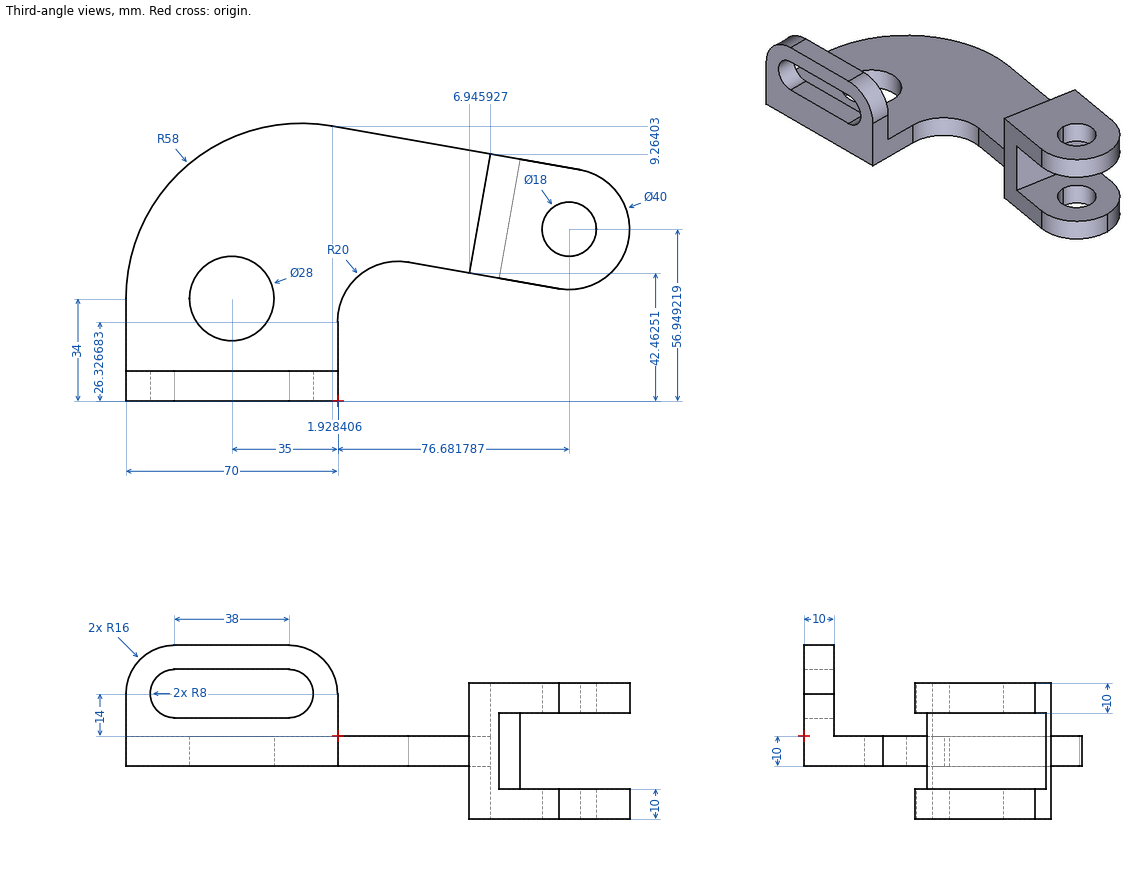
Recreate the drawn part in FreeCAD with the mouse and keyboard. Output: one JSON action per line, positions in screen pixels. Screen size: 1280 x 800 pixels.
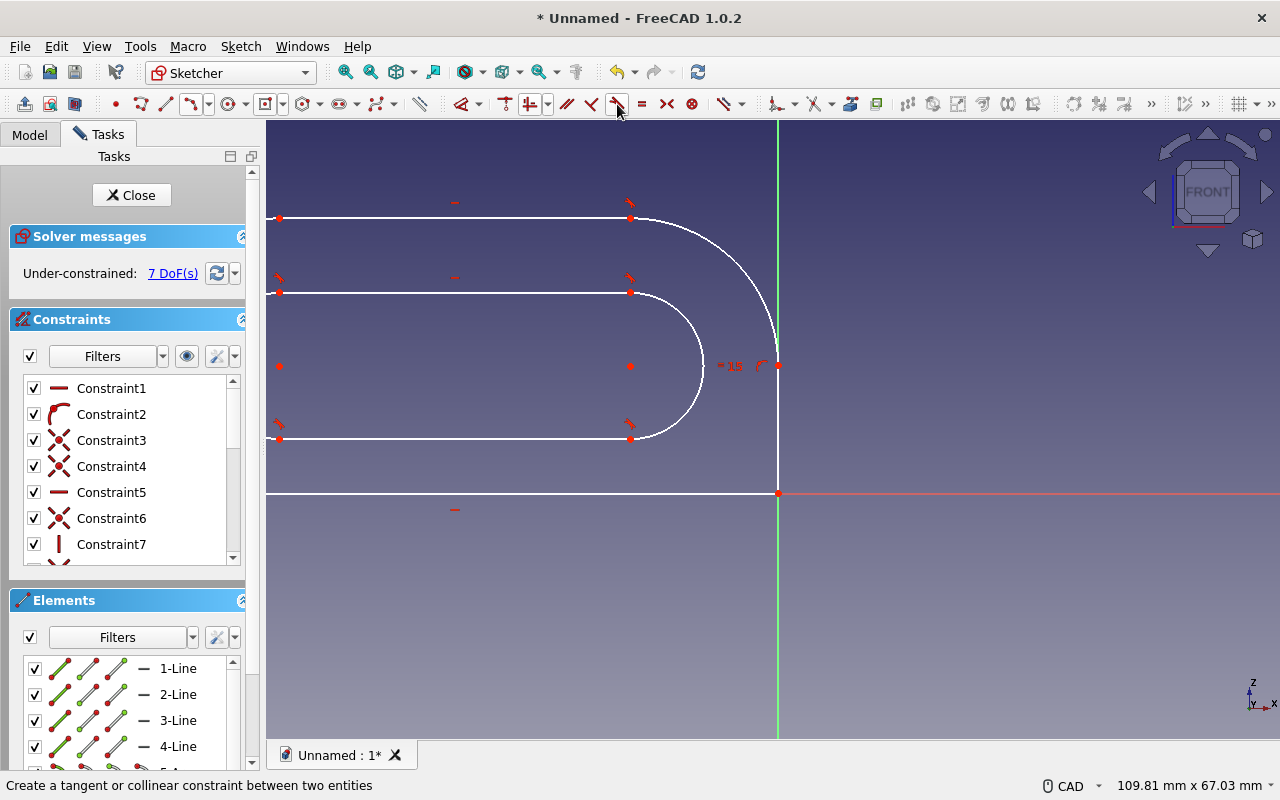
{"action": "left_click", "coordinate": [385, 218]}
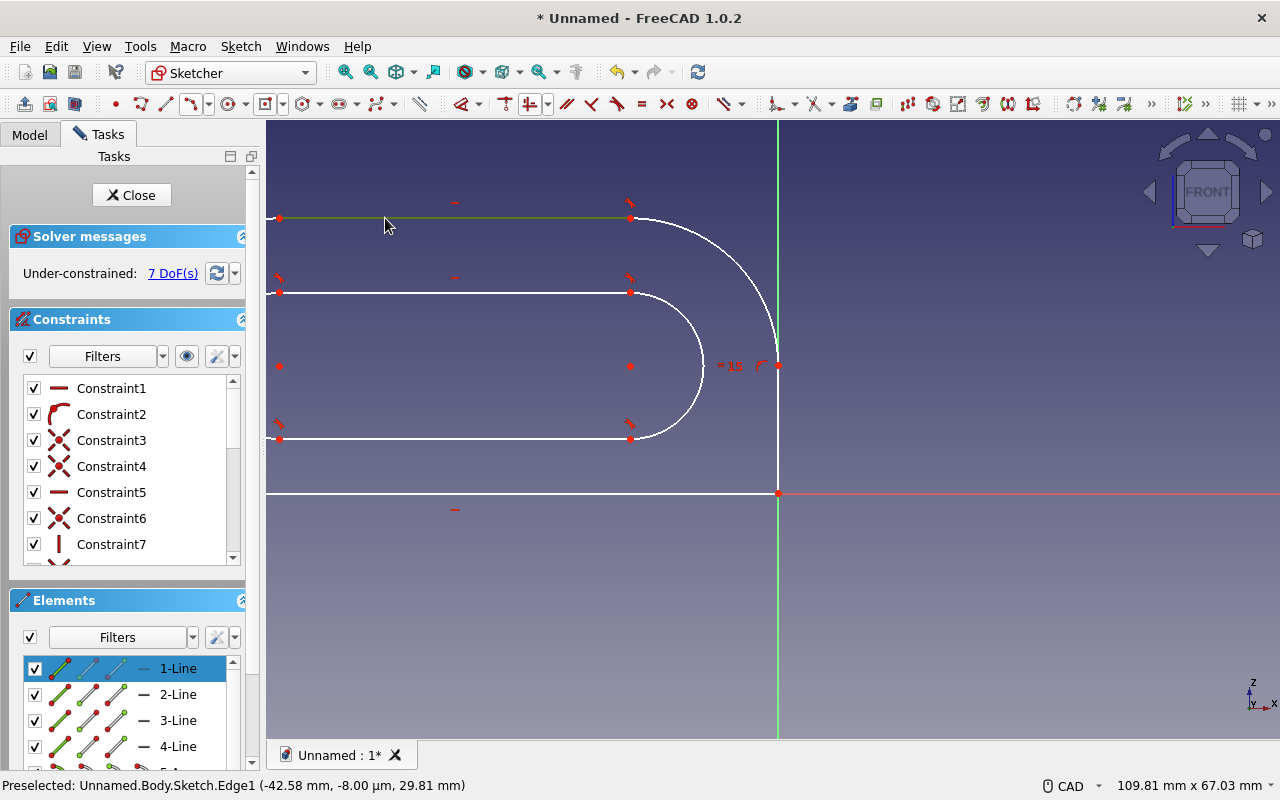
{"action": "scroll", "coordinate": [1115, 581], "scroll_direction": "down", "scroll_amount": 2}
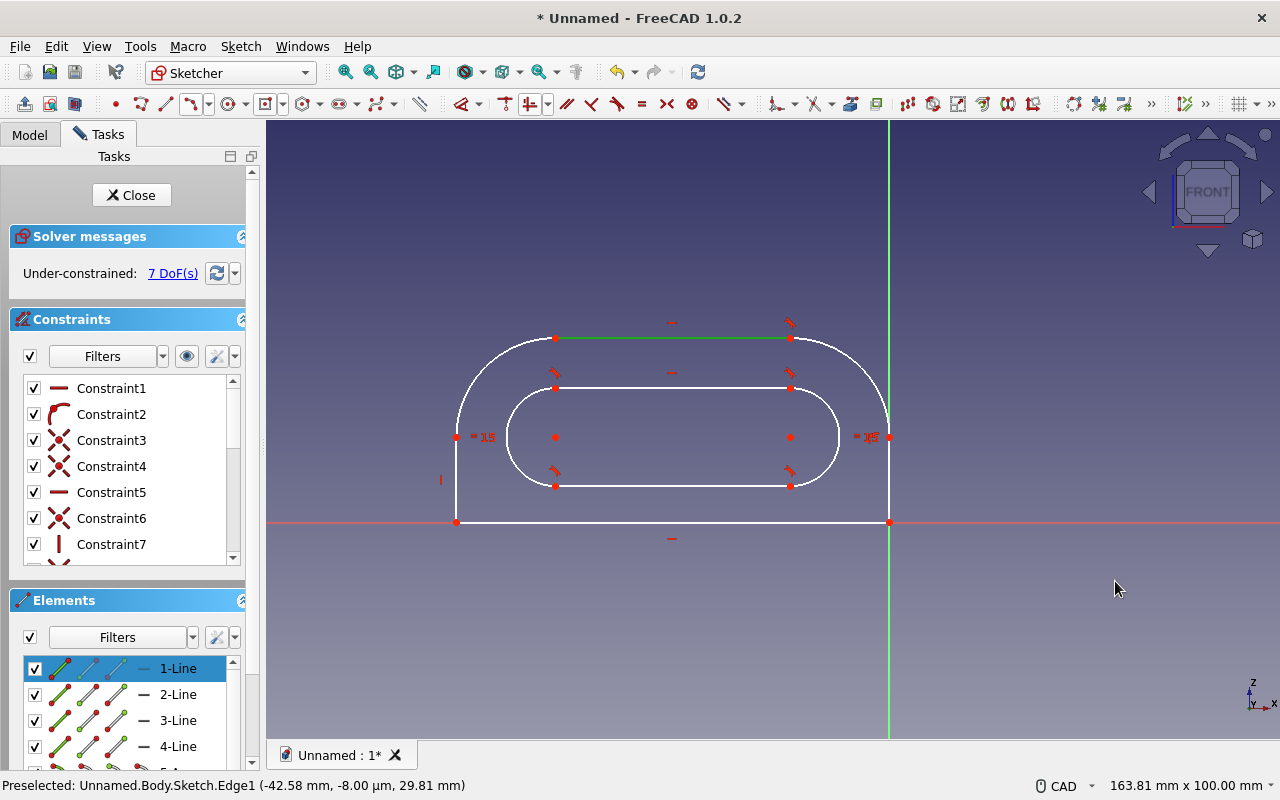
{"action": "left_click", "coordinate": [511, 349]}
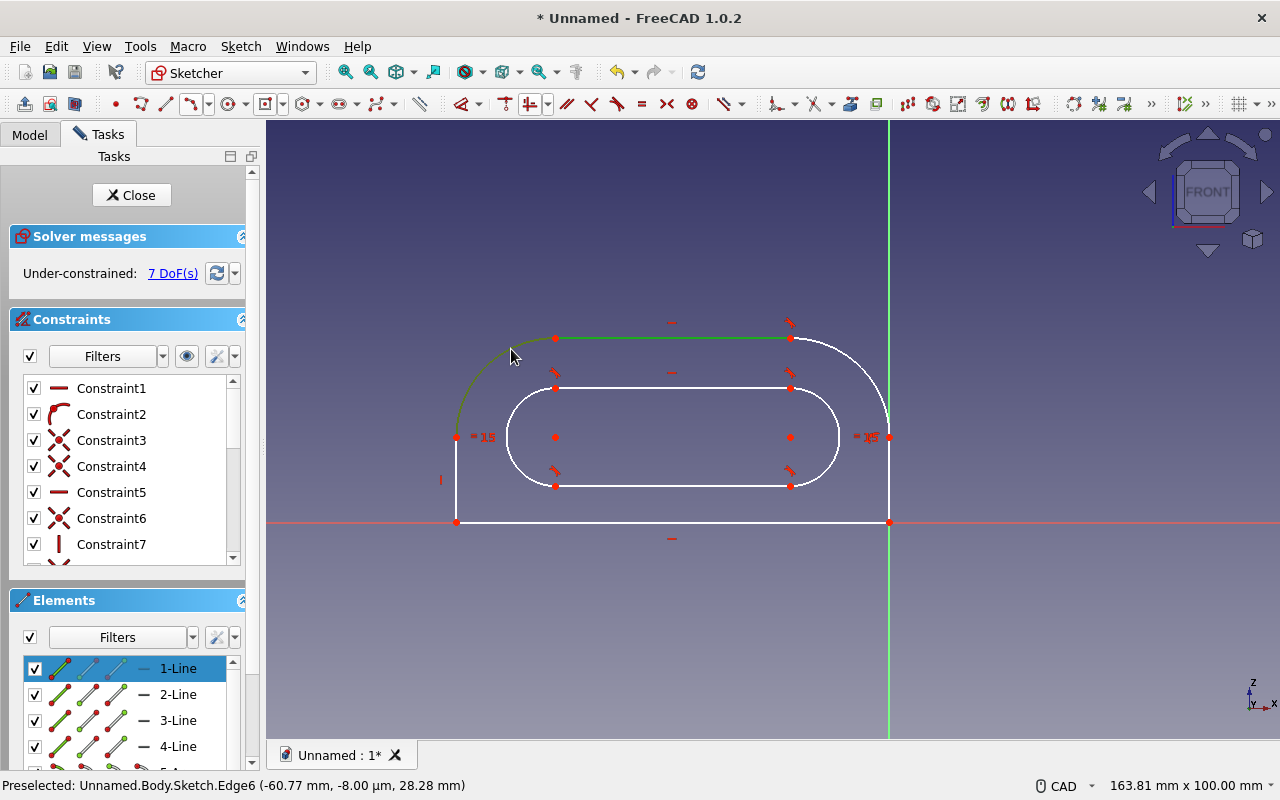
{"action": "left_click", "coordinate": [617, 104]}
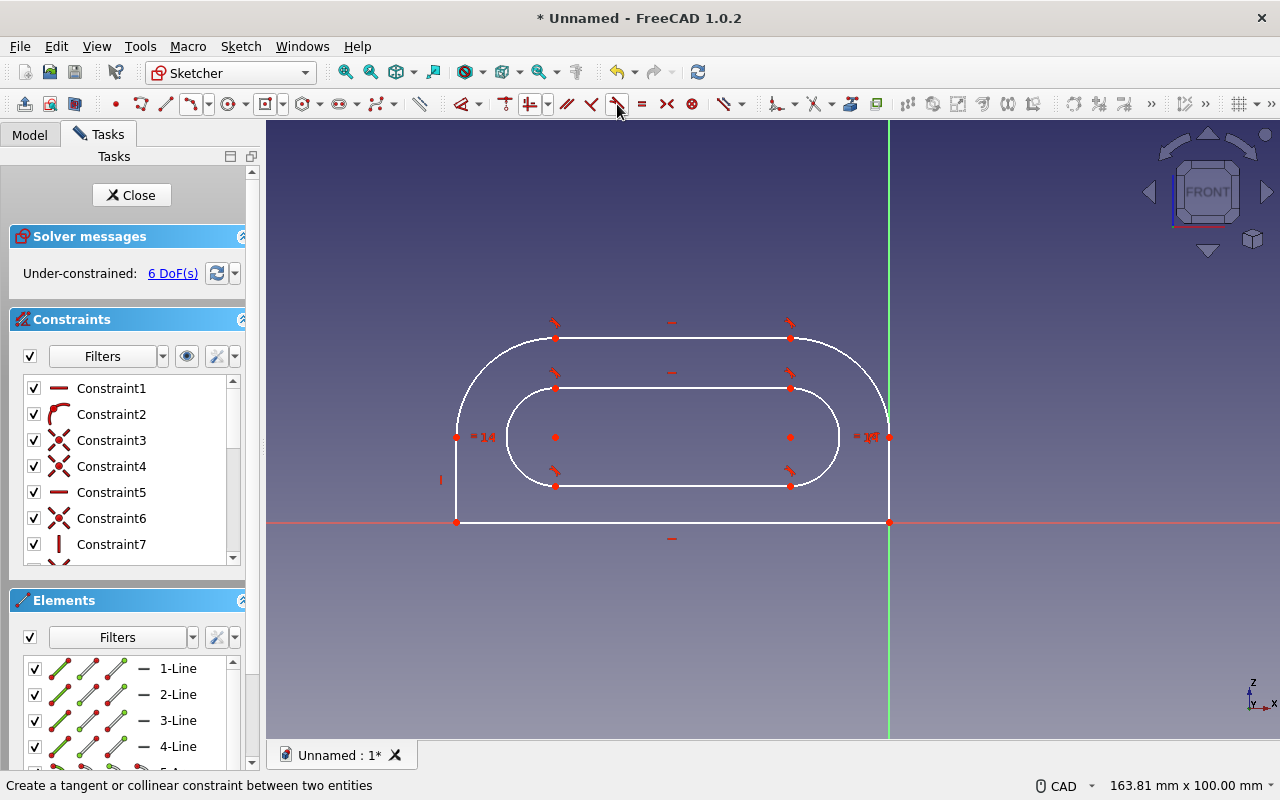
{"action": "left_click", "coordinate": [889, 463]}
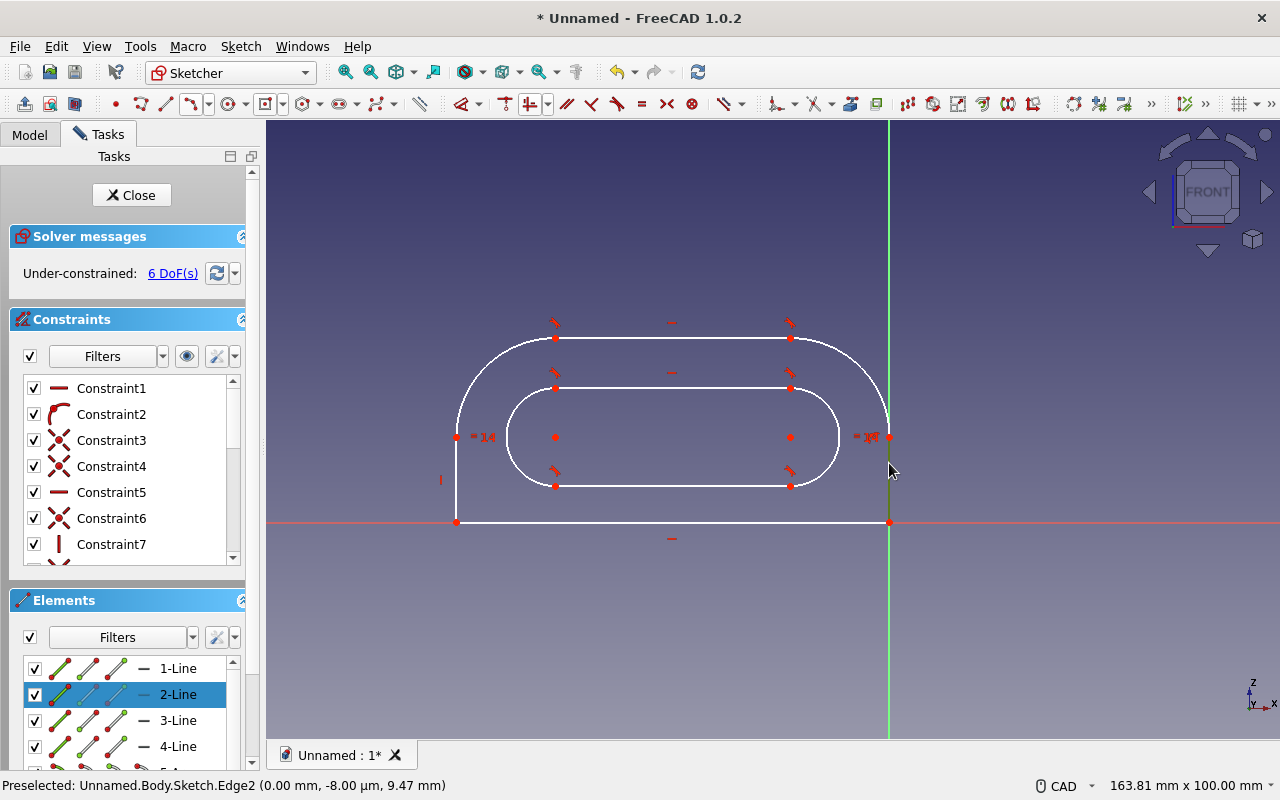
{"action": "scroll", "coordinate": [879, 392], "scroll_direction": "up", "scroll_amount": 2}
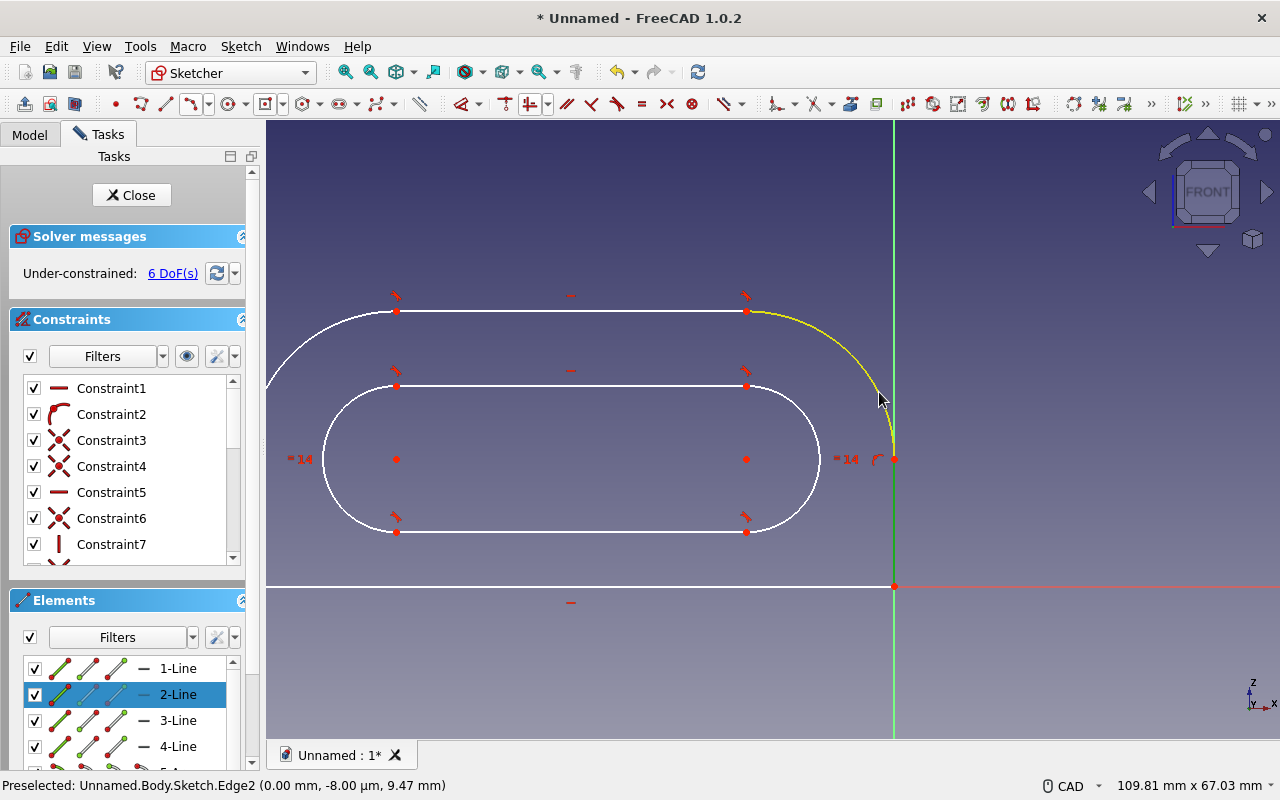
{"action": "left_click", "coordinate": [878, 392]}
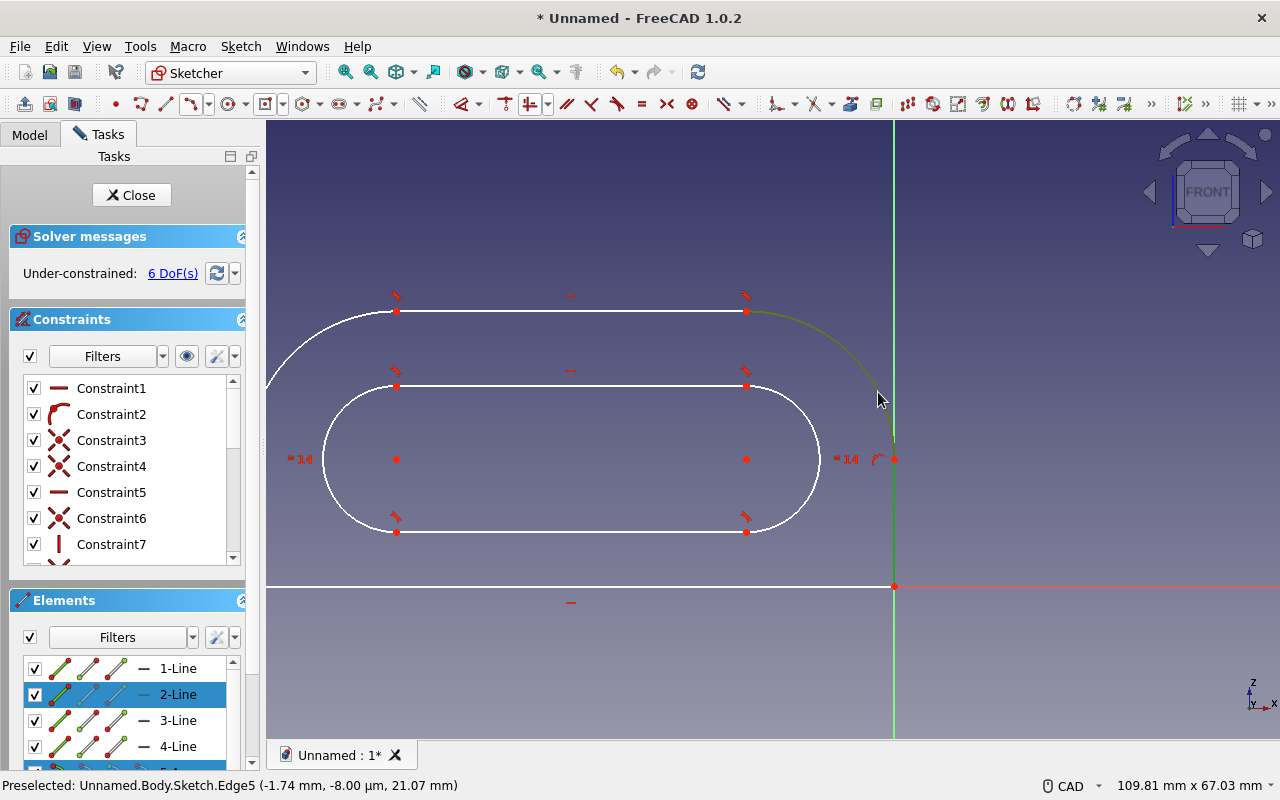
{"action": "left_click", "coordinate": [617, 104]}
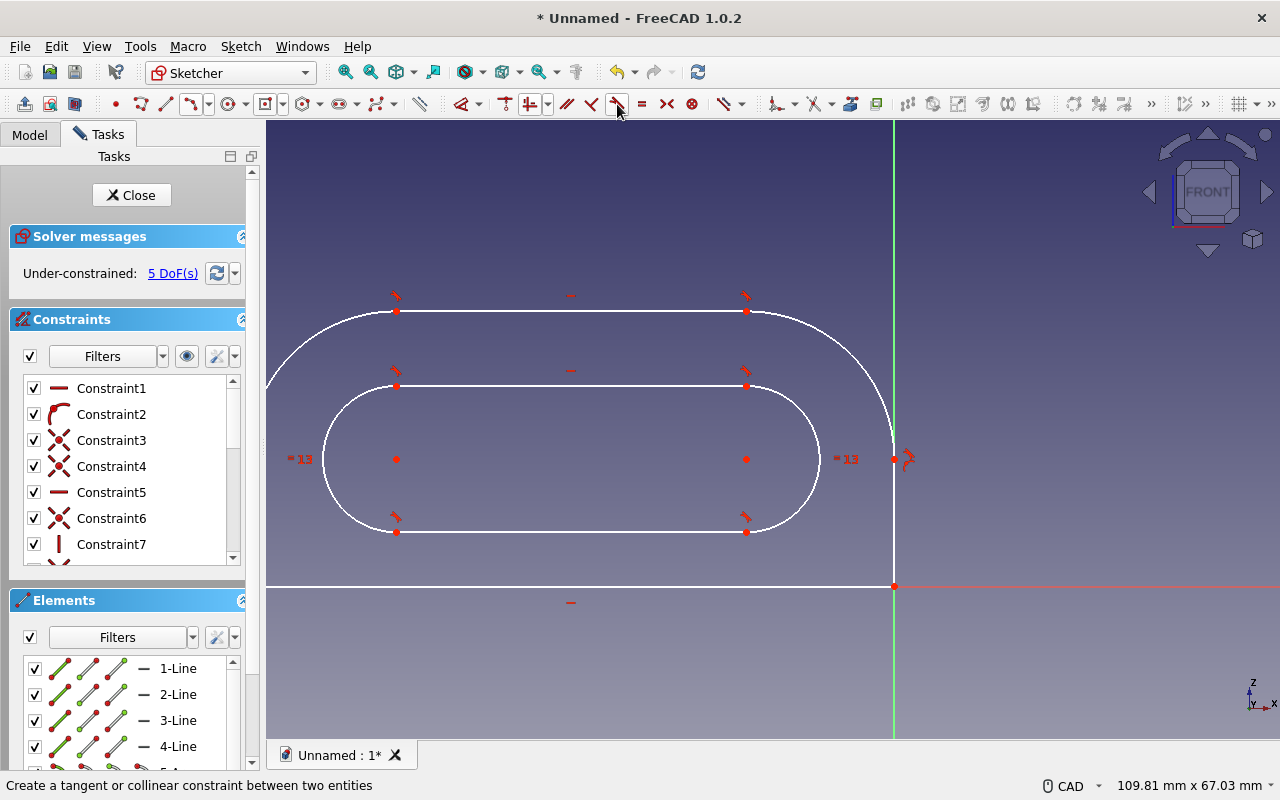
{"action": "scroll", "coordinate": [1115, 345], "scroll_direction": "down", "scroll_amount": 1}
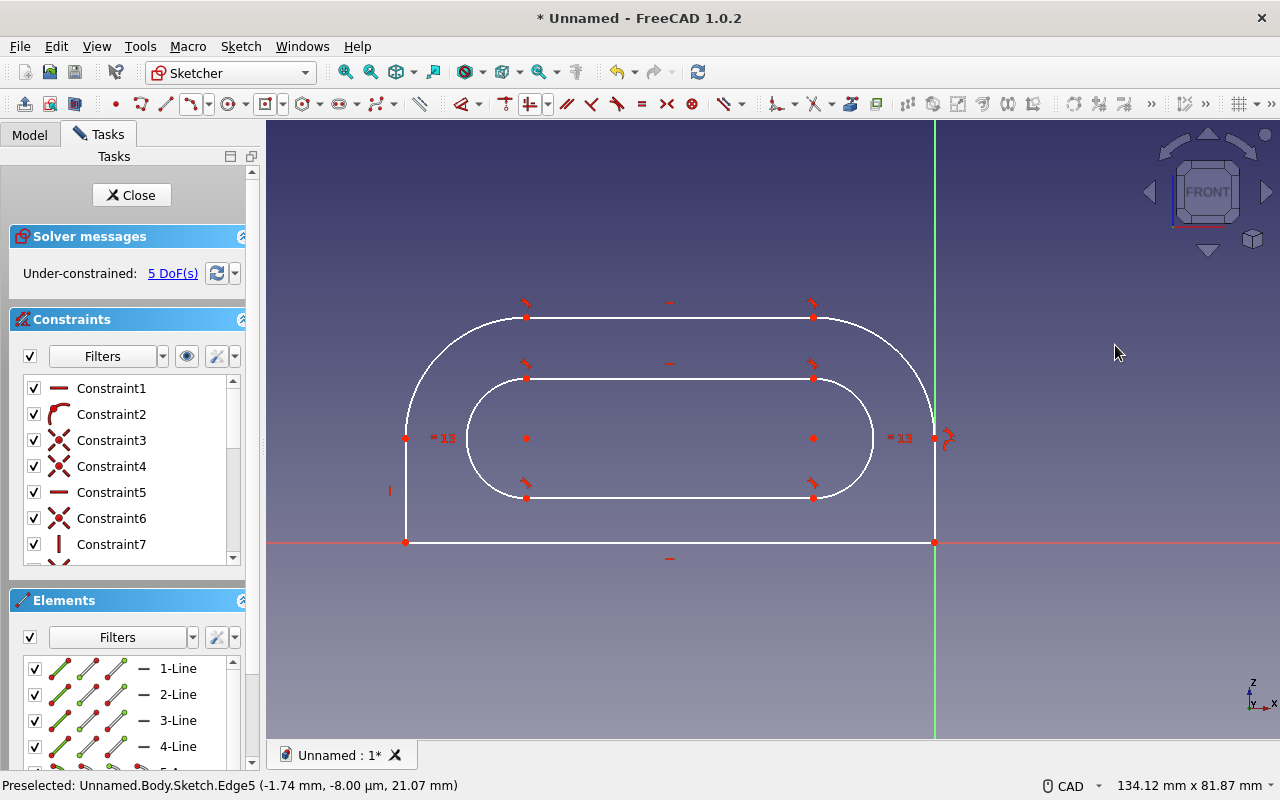
{"action": "left_click", "coordinate": [406, 512]}